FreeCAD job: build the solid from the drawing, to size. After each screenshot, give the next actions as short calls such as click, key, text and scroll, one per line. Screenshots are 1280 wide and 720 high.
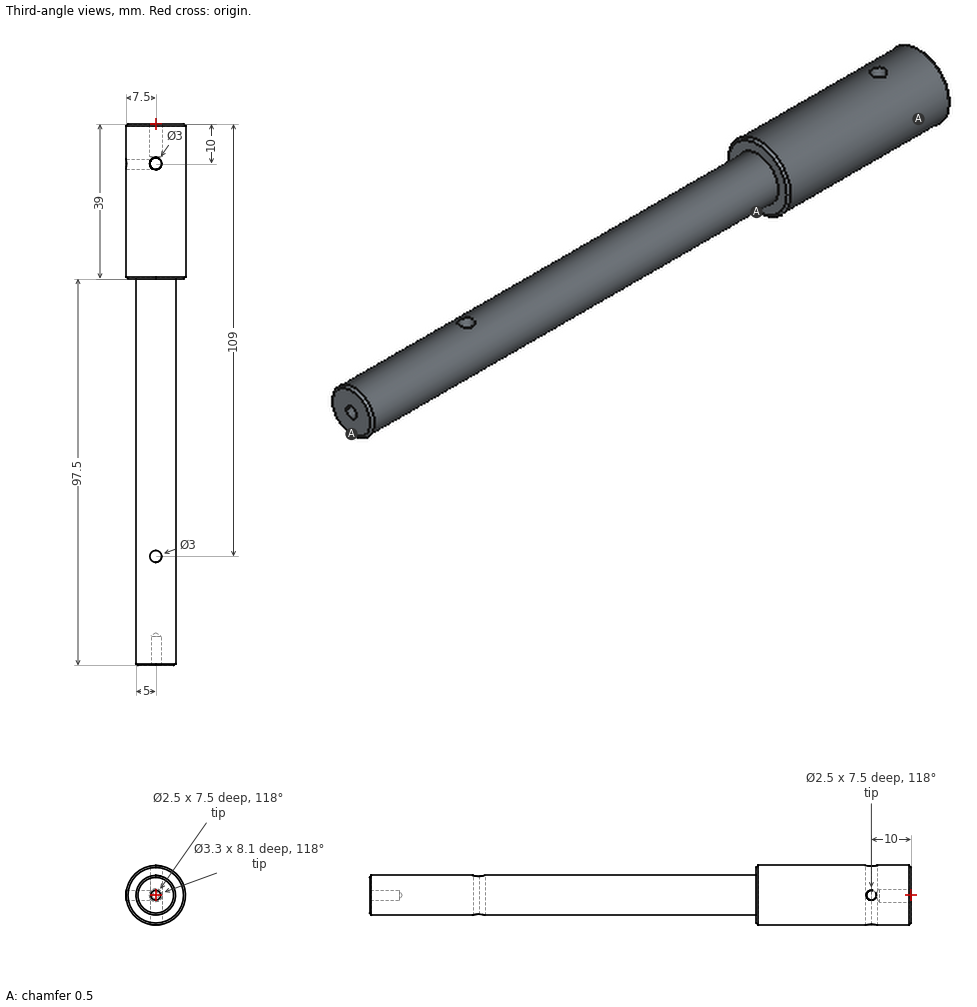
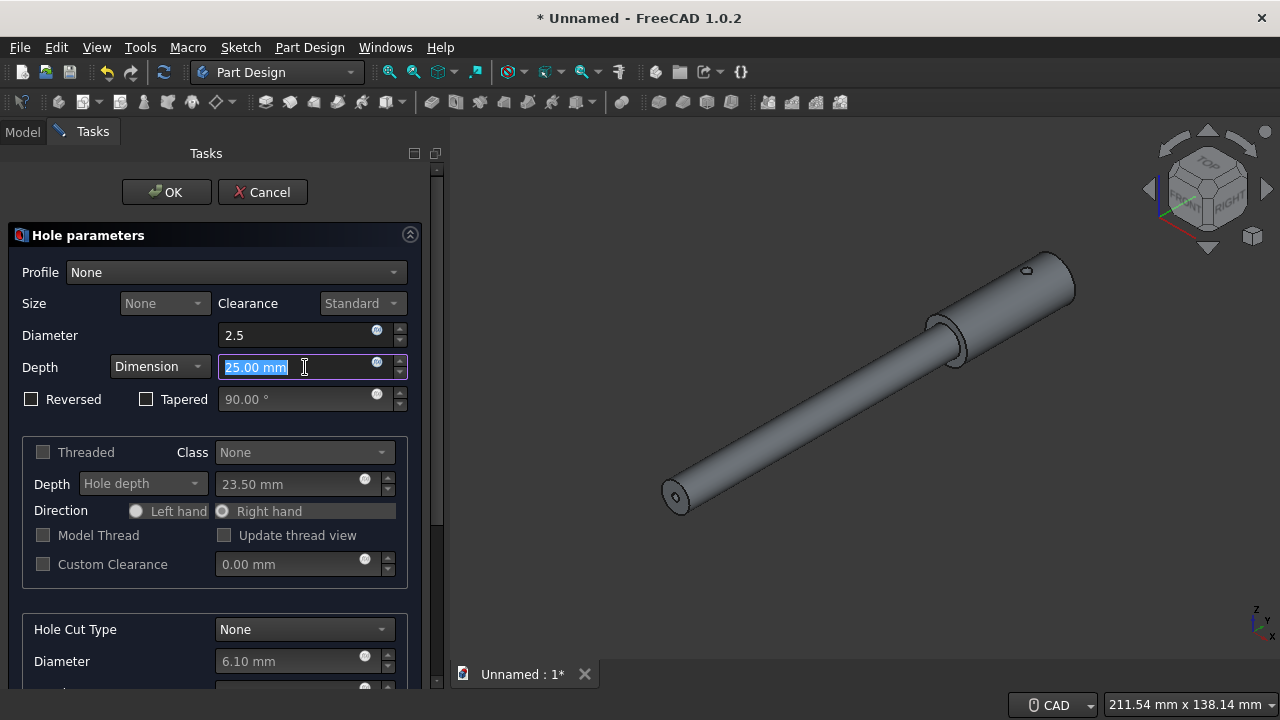
text(7.5)
key(Tab)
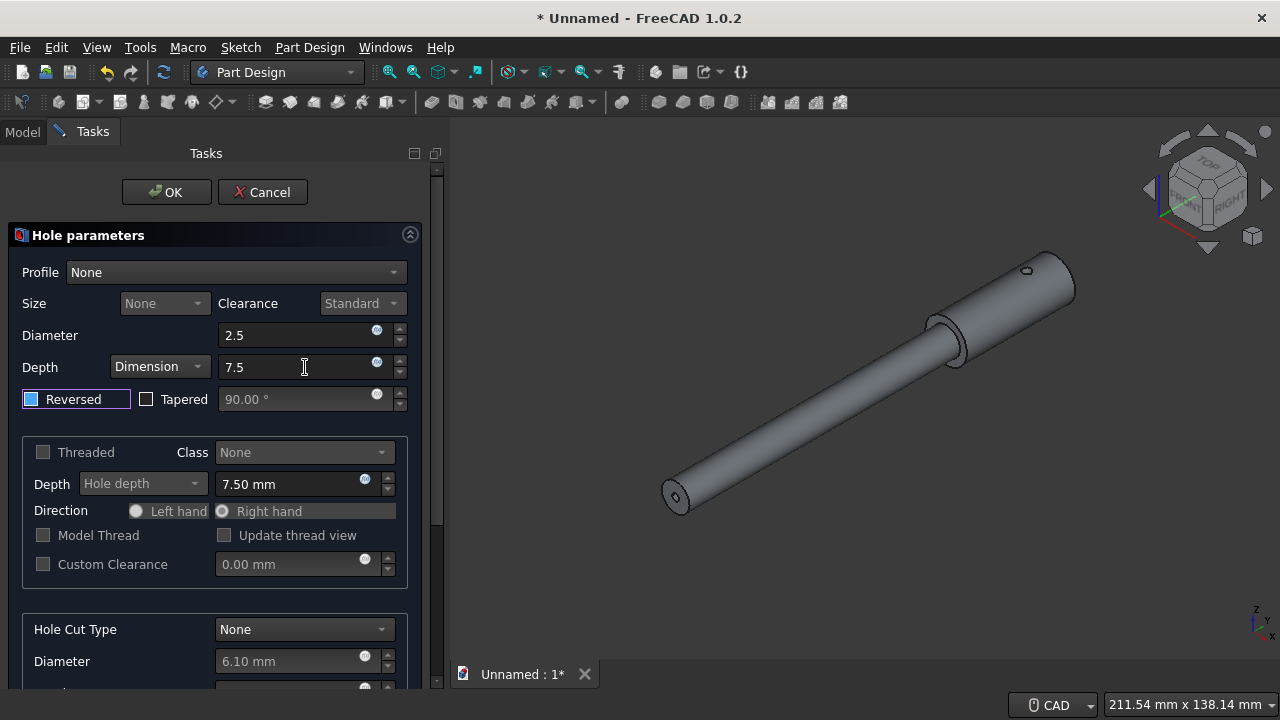
click(167, 192)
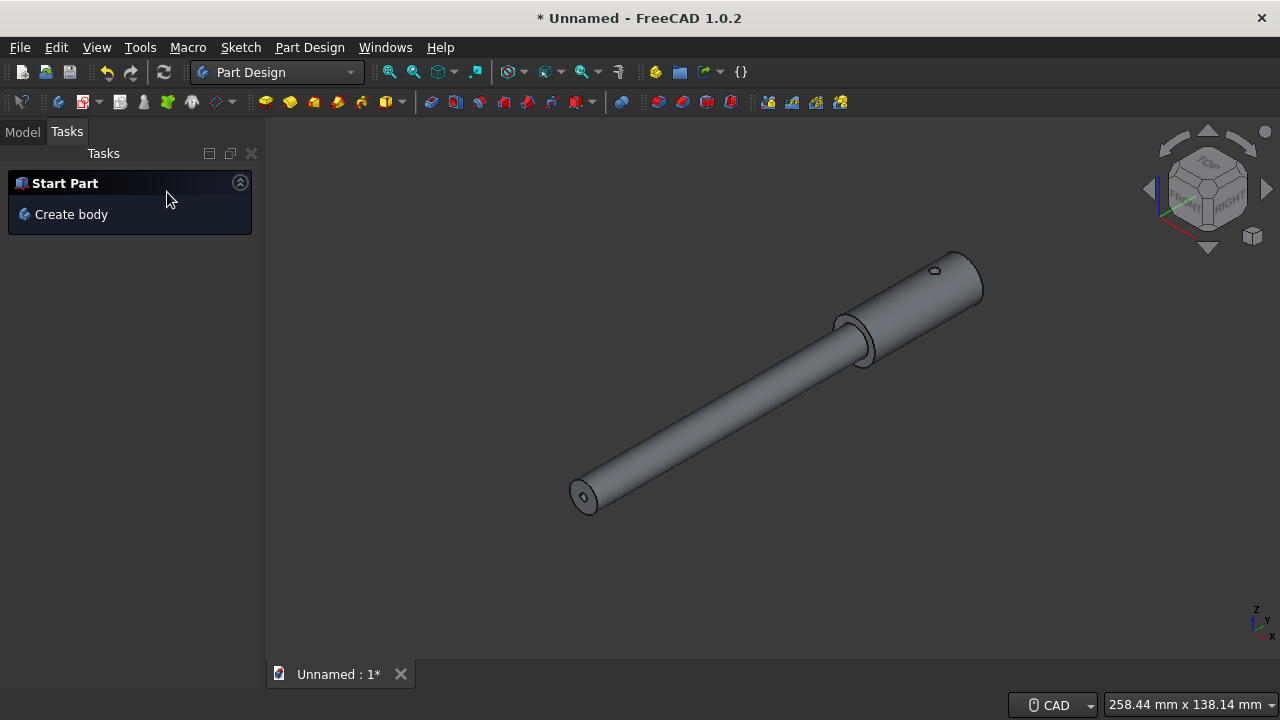
click(598, 504)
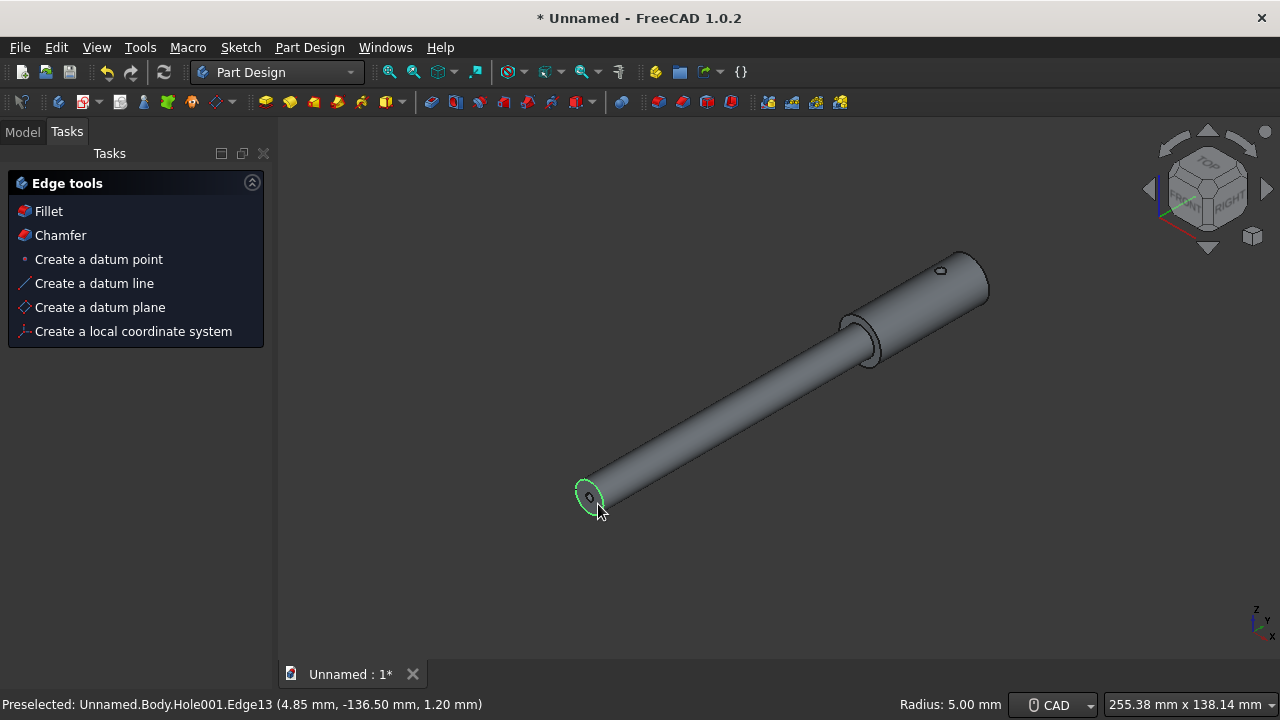
click(881, 352, ctrl)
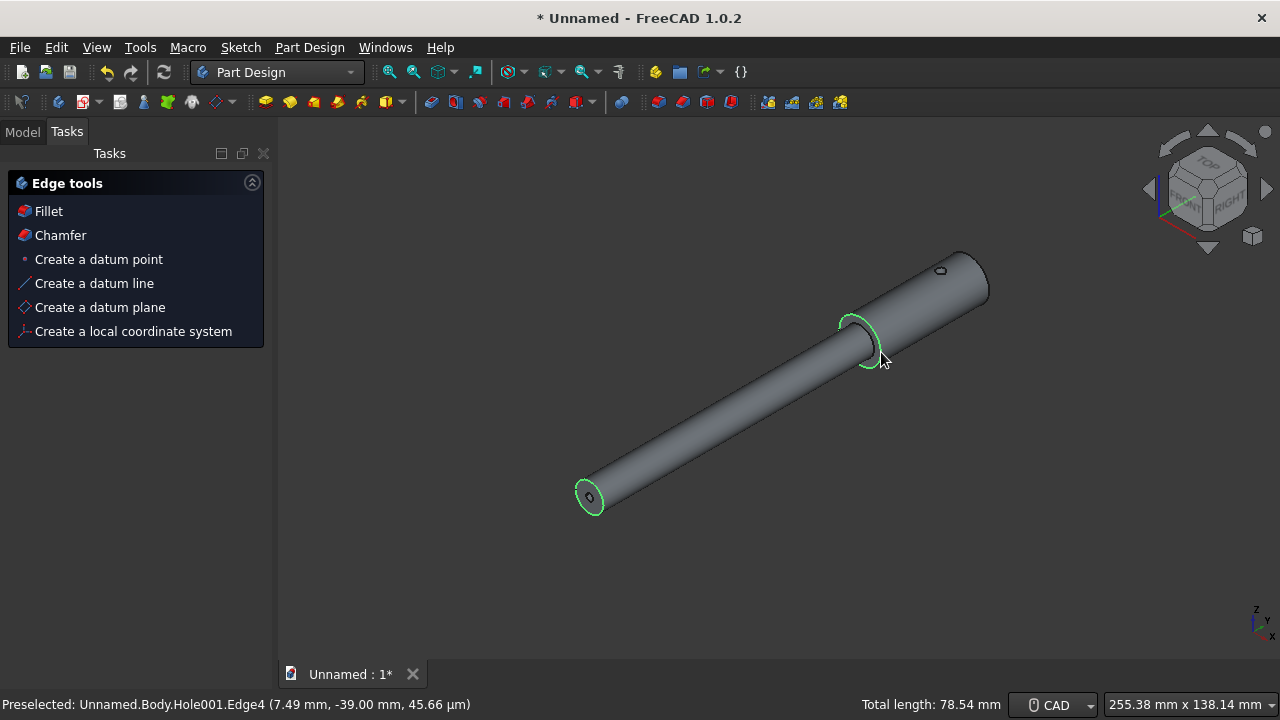
key(2)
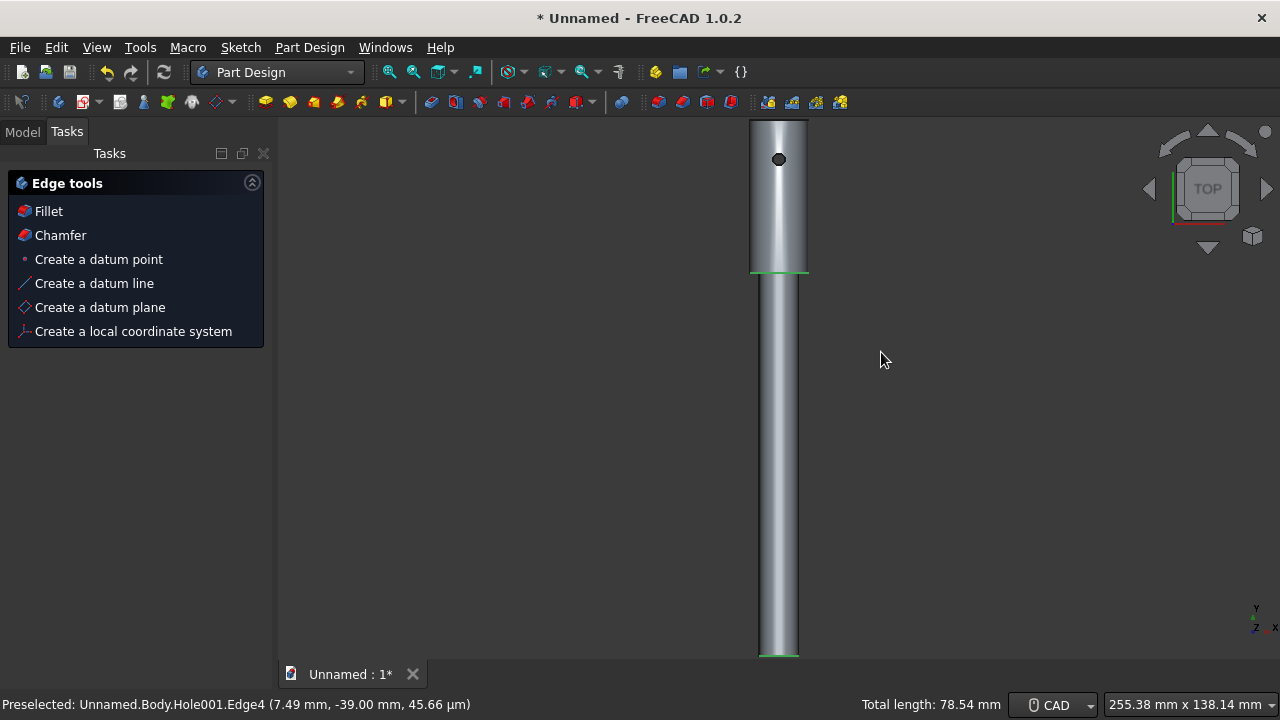
key(0)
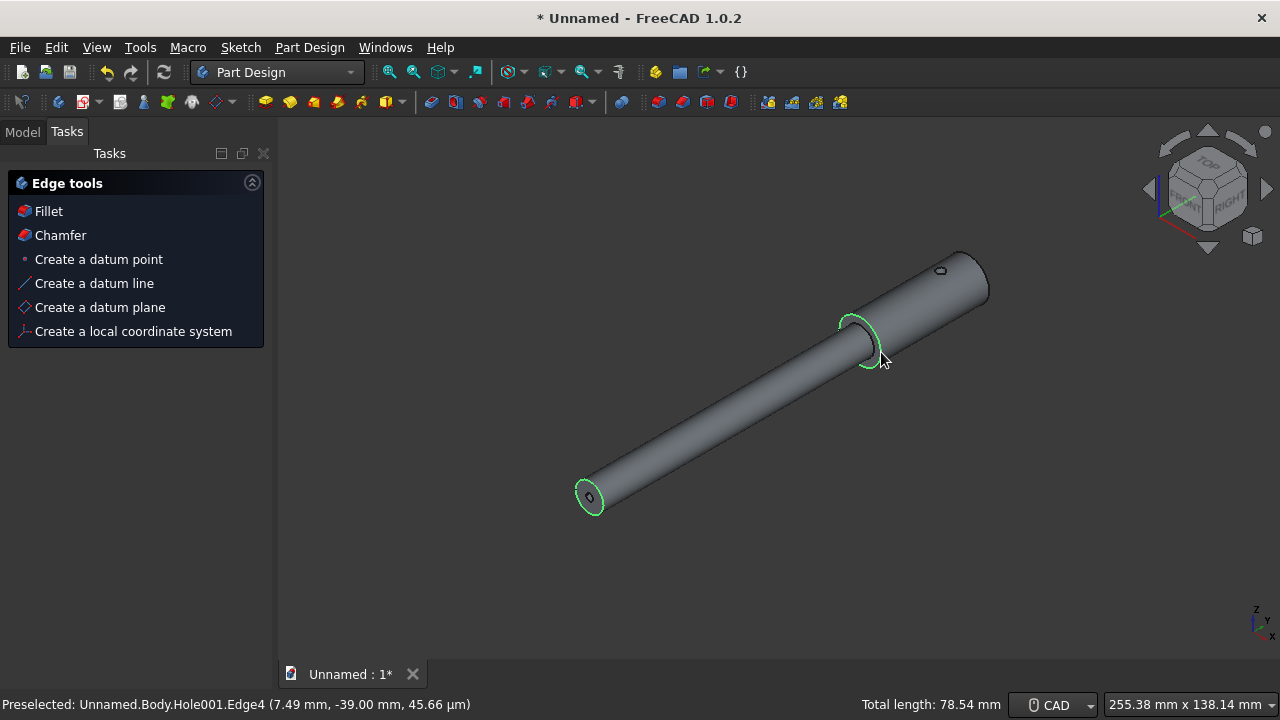
key(1)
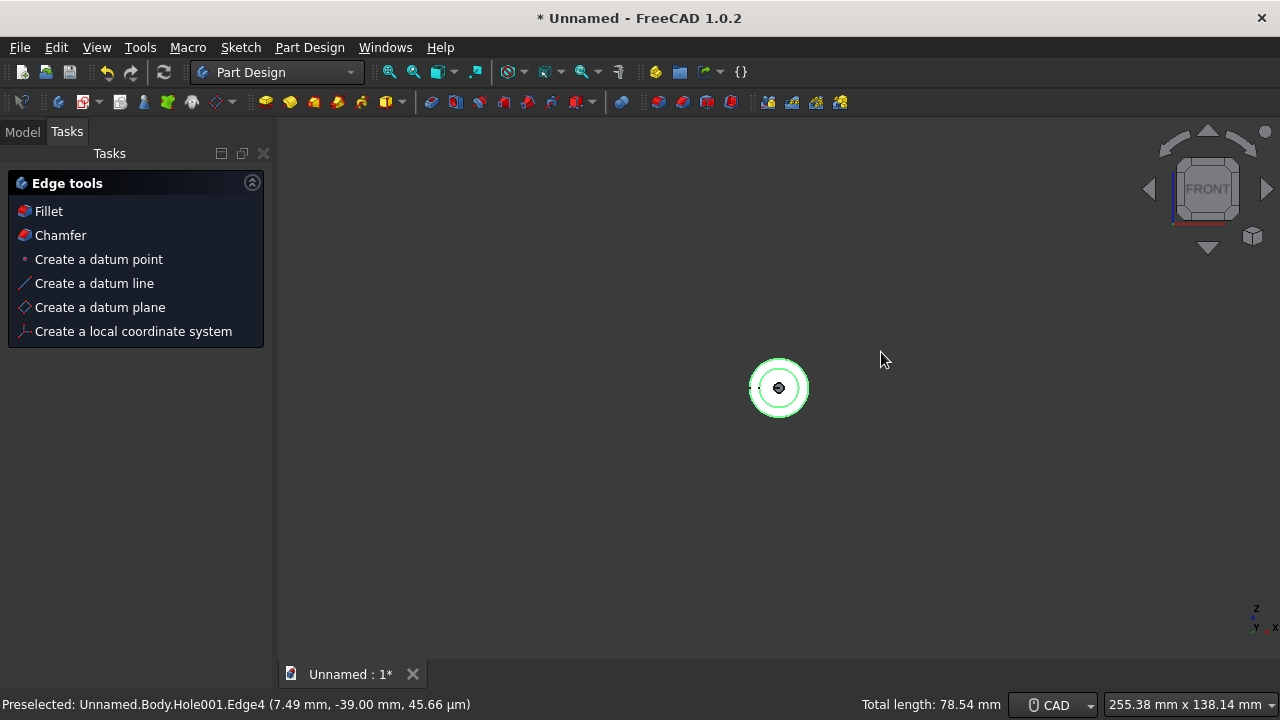
click(390, 72)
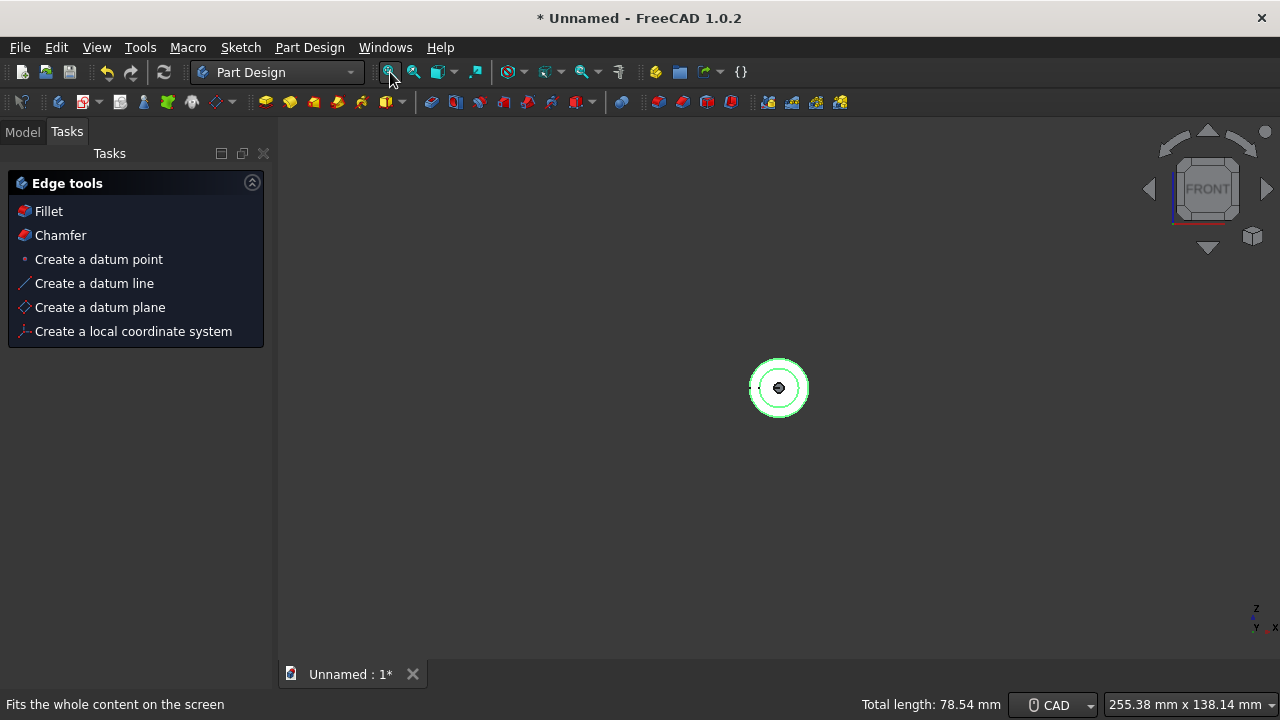
key(3)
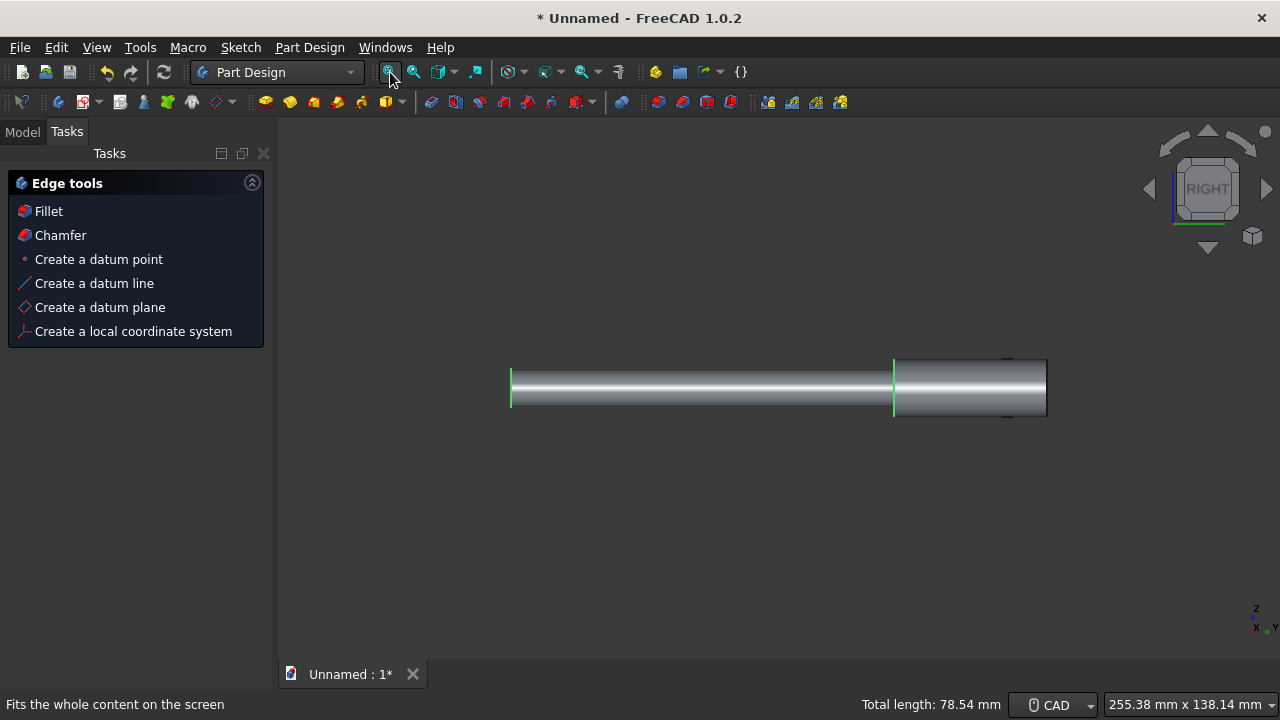
click(1047, 387, ctrl)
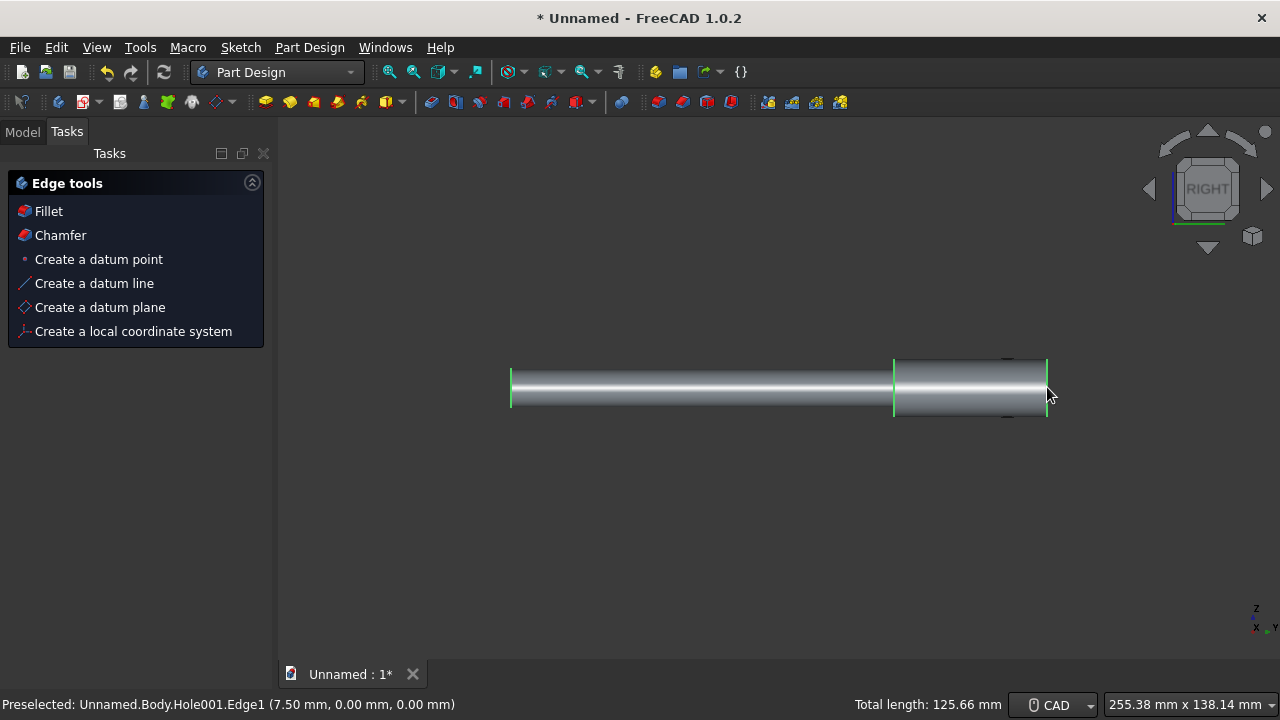
click(684, 102)